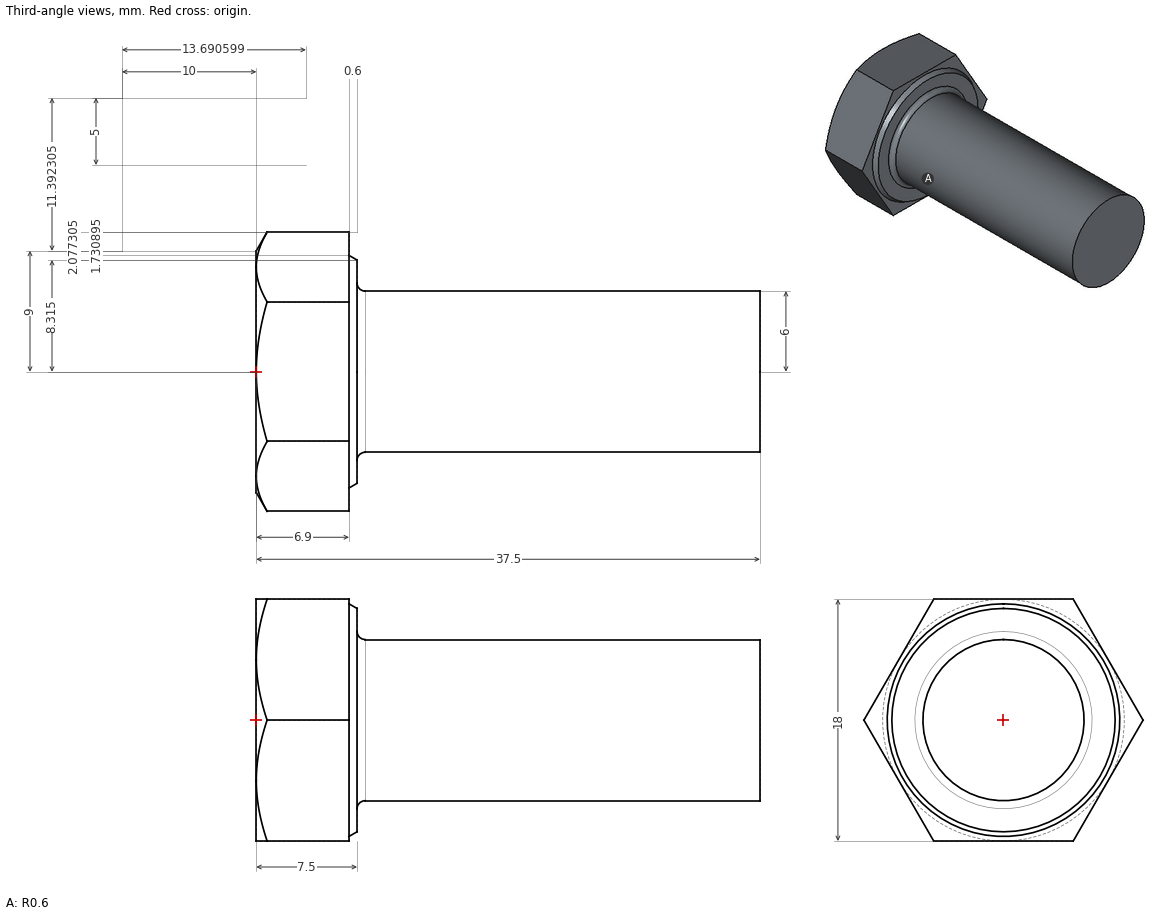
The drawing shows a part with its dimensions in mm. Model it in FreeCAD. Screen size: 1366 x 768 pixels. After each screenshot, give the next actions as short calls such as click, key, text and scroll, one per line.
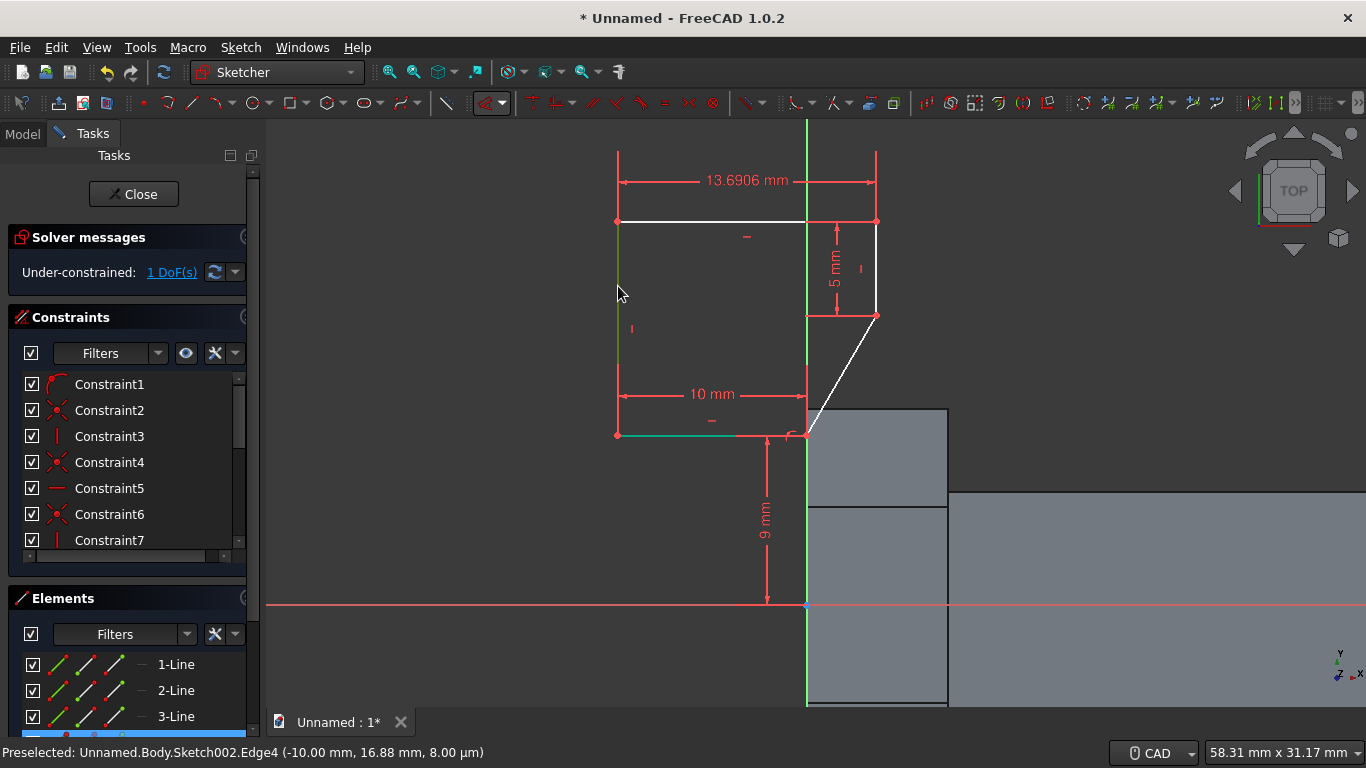
click(504, 104)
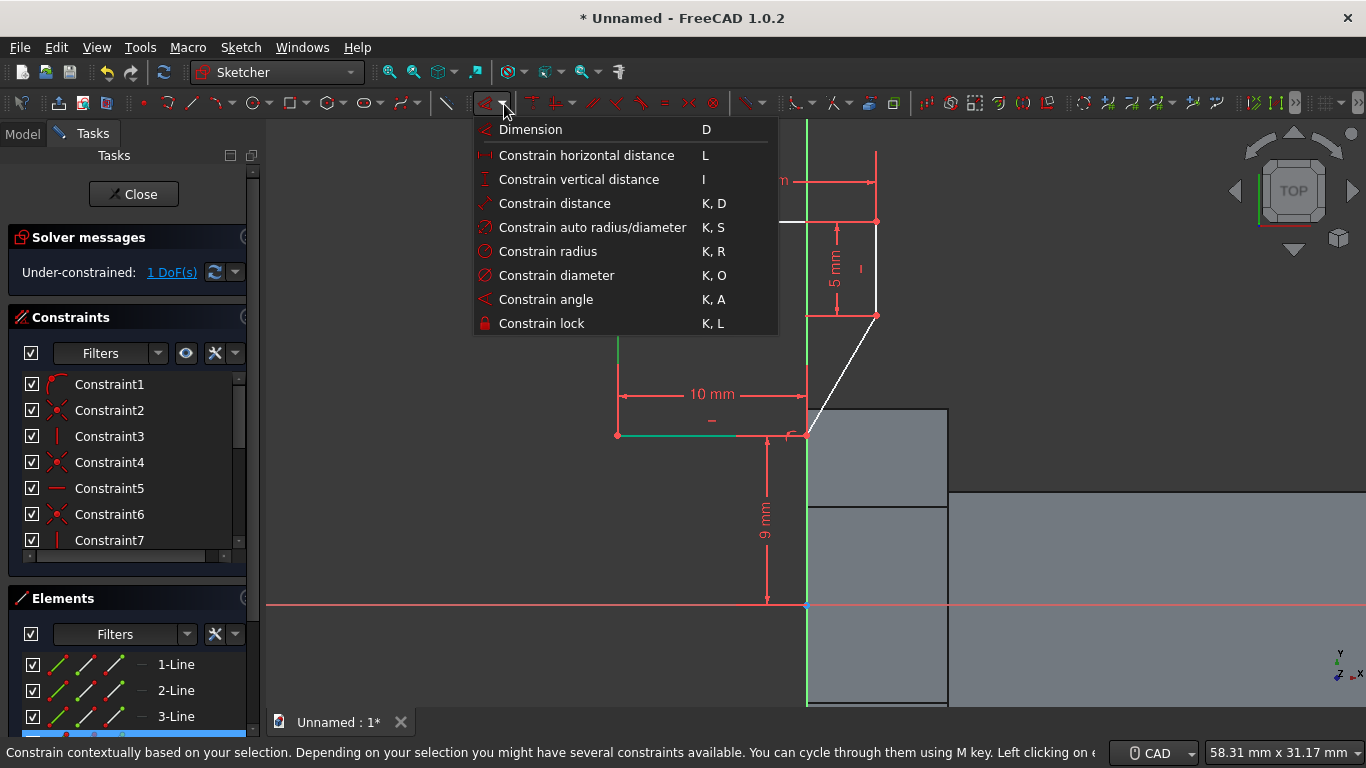
click(626, 179)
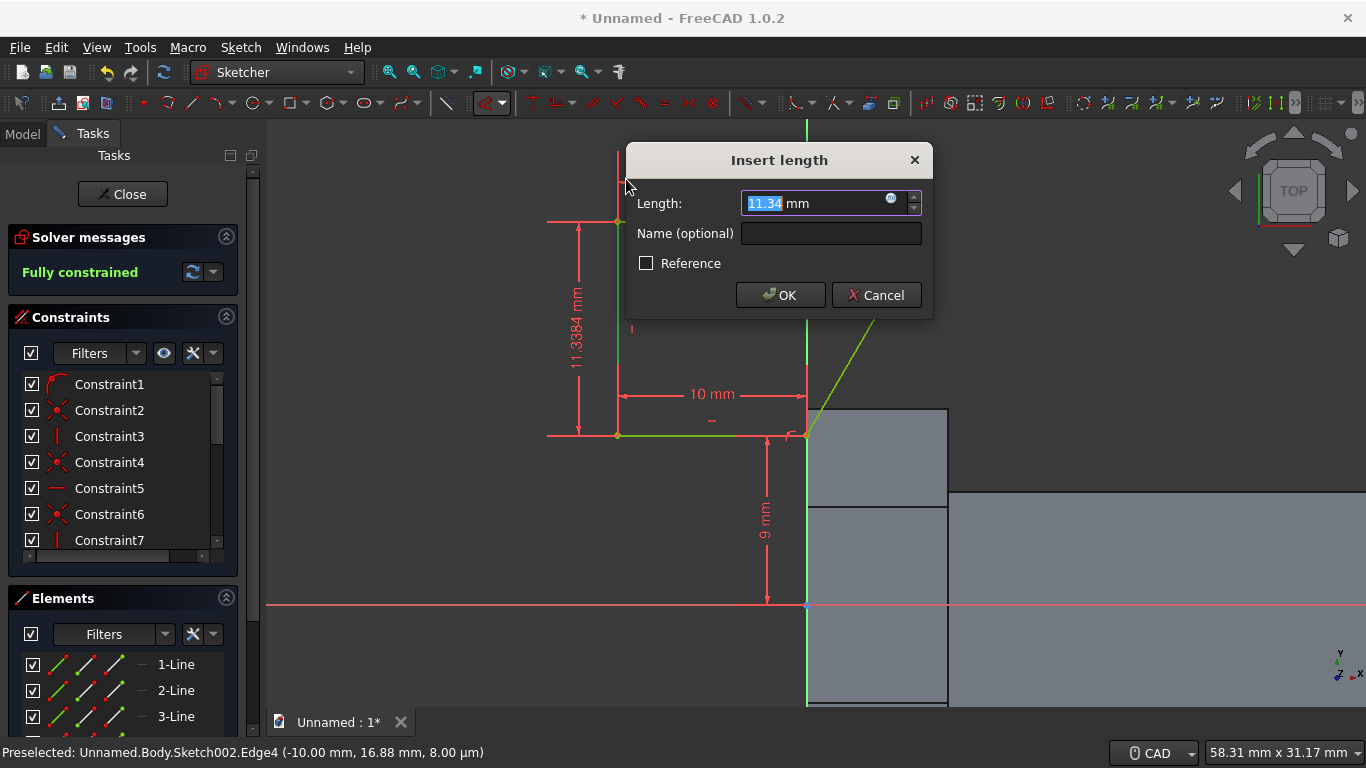
text(11.392305)
key(Return)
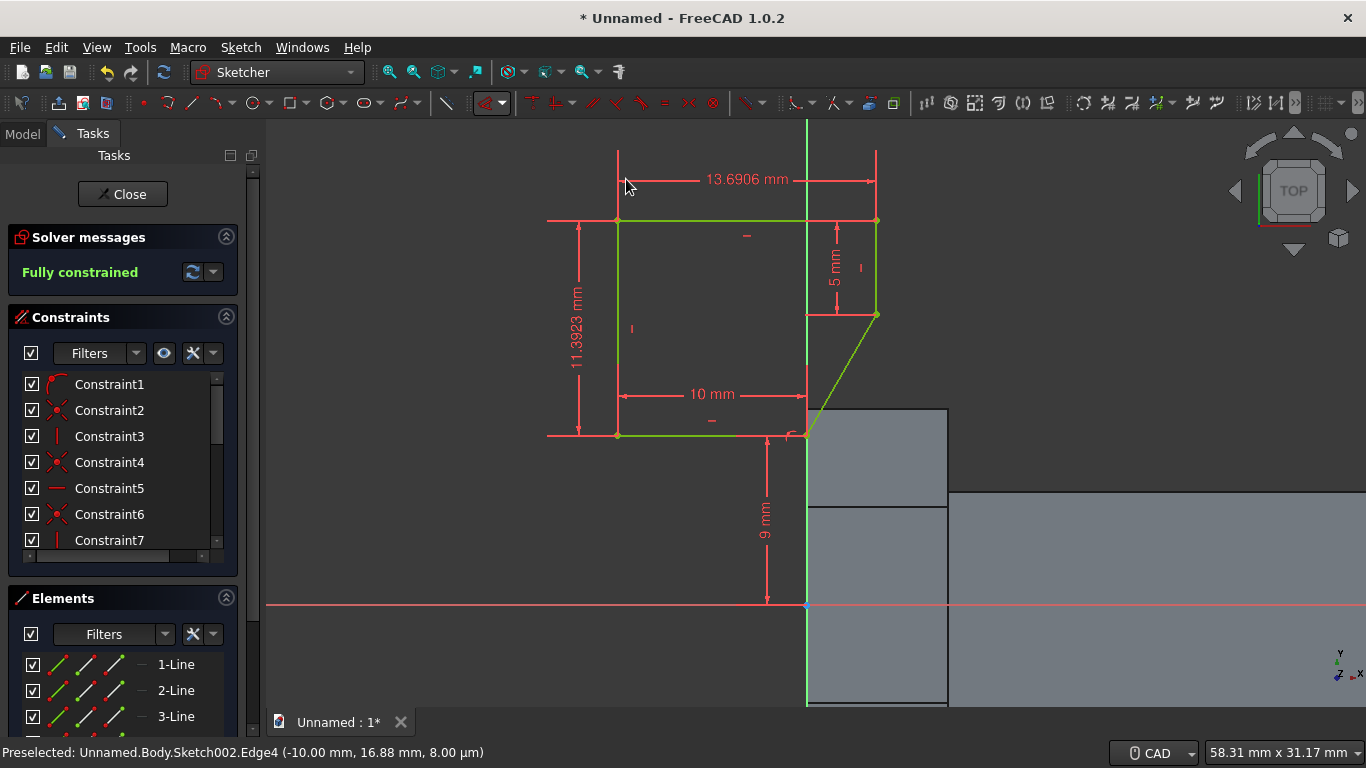
click(123, 194)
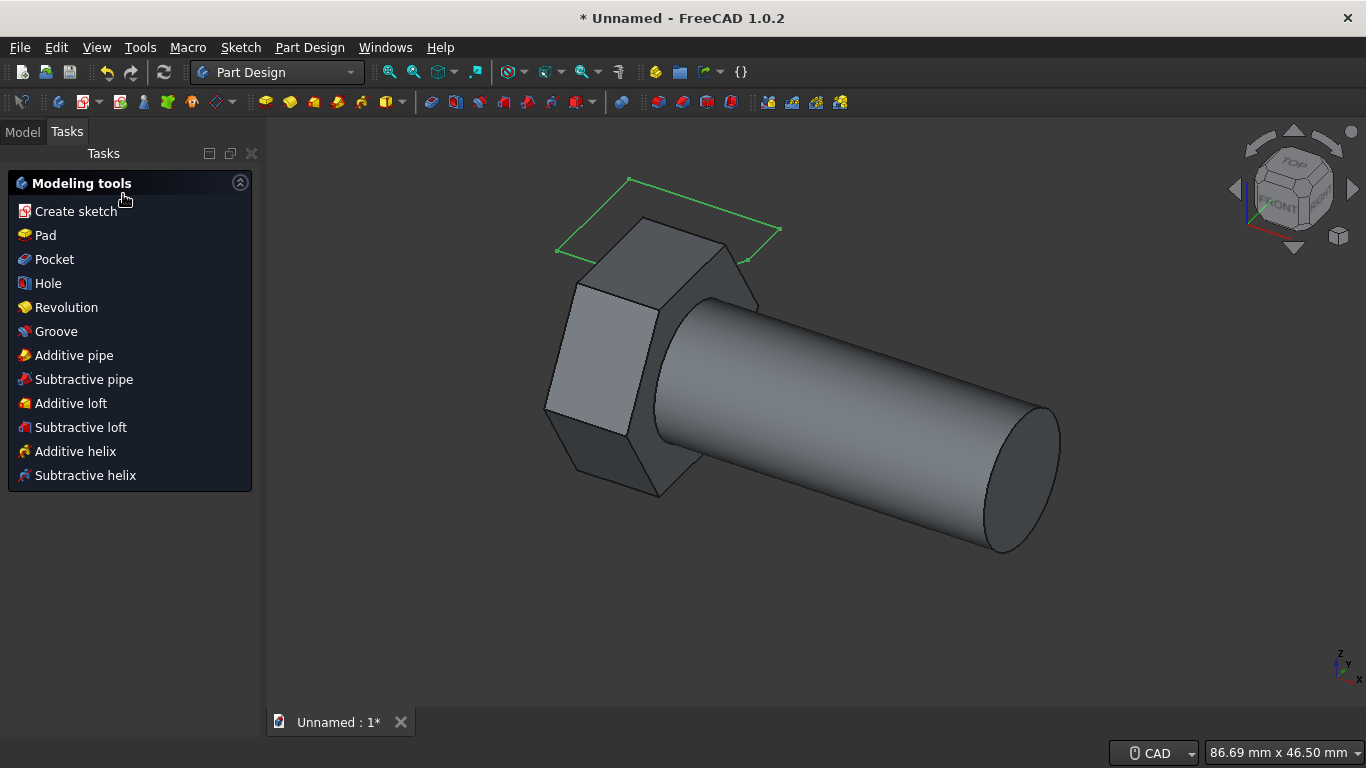
click(480, 102)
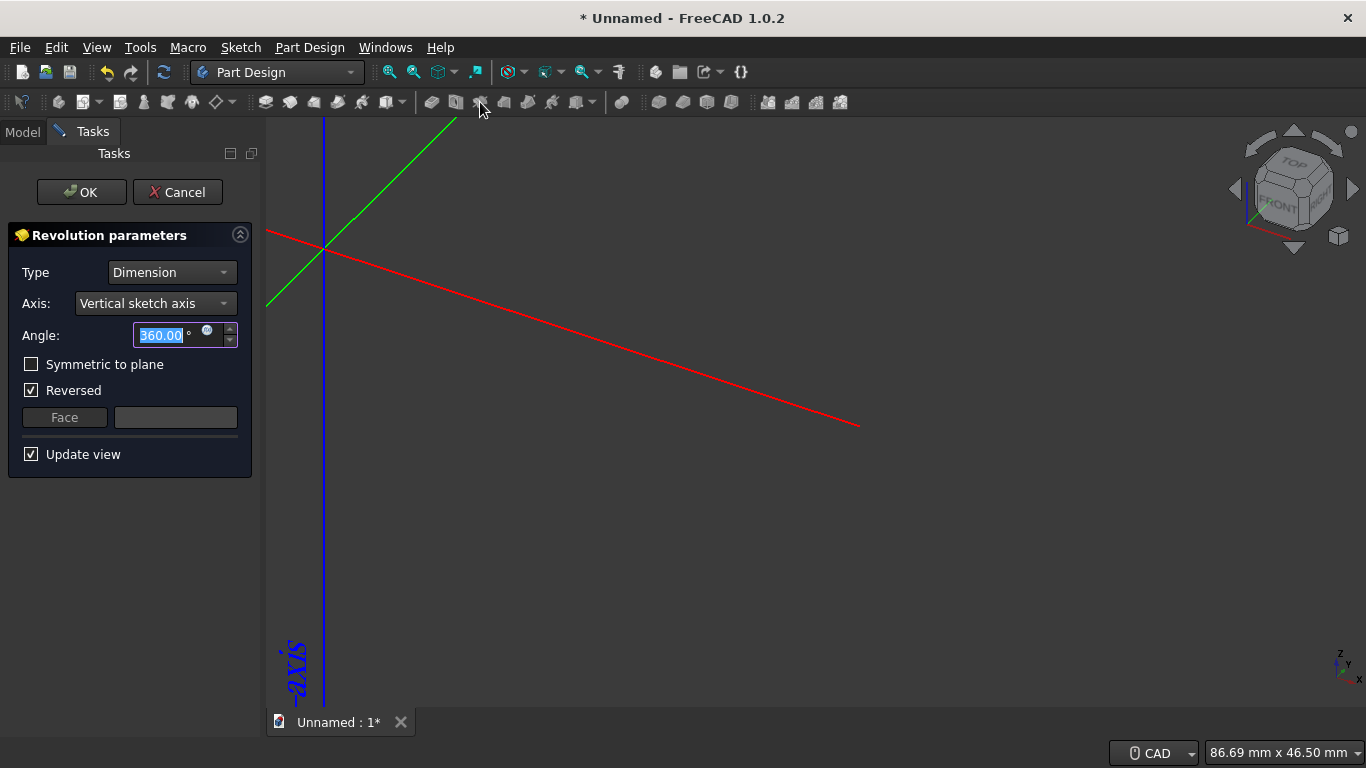
click(156, 304)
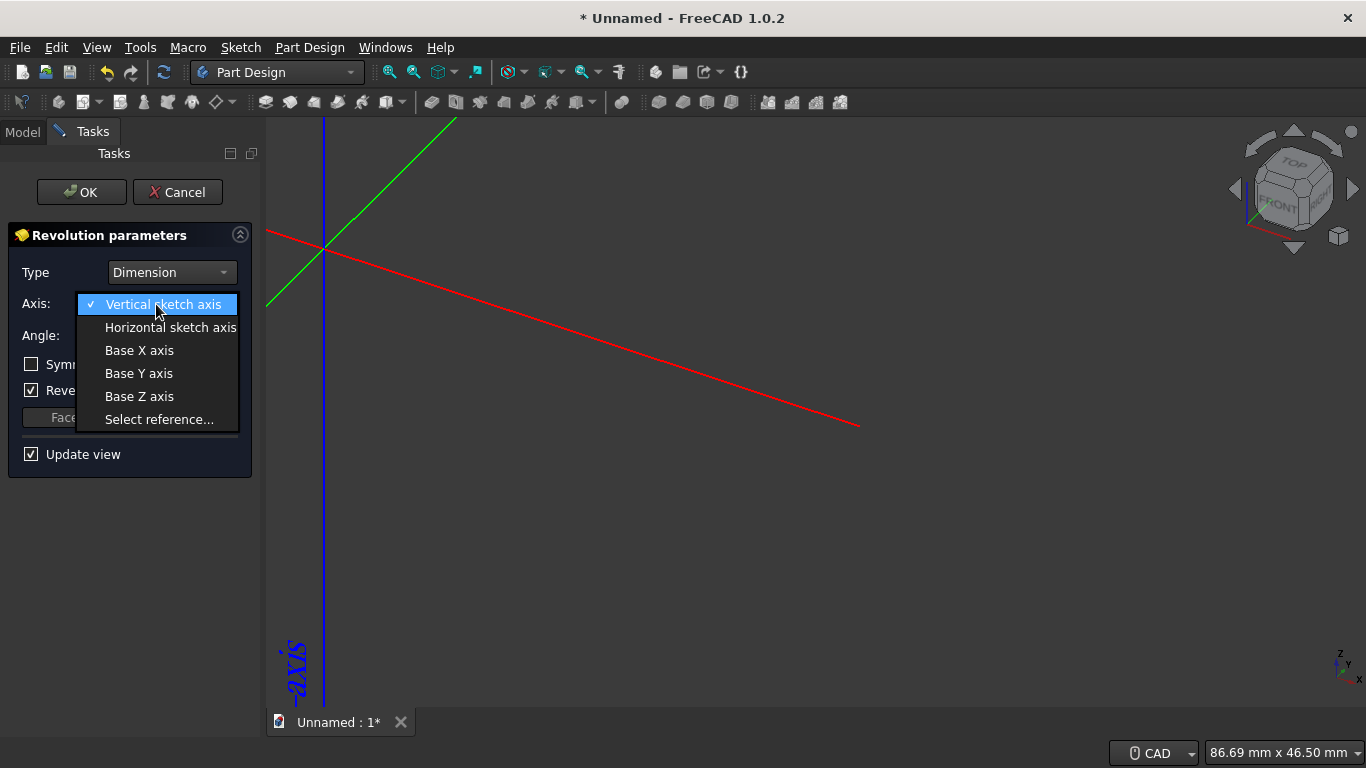
click(156, 328)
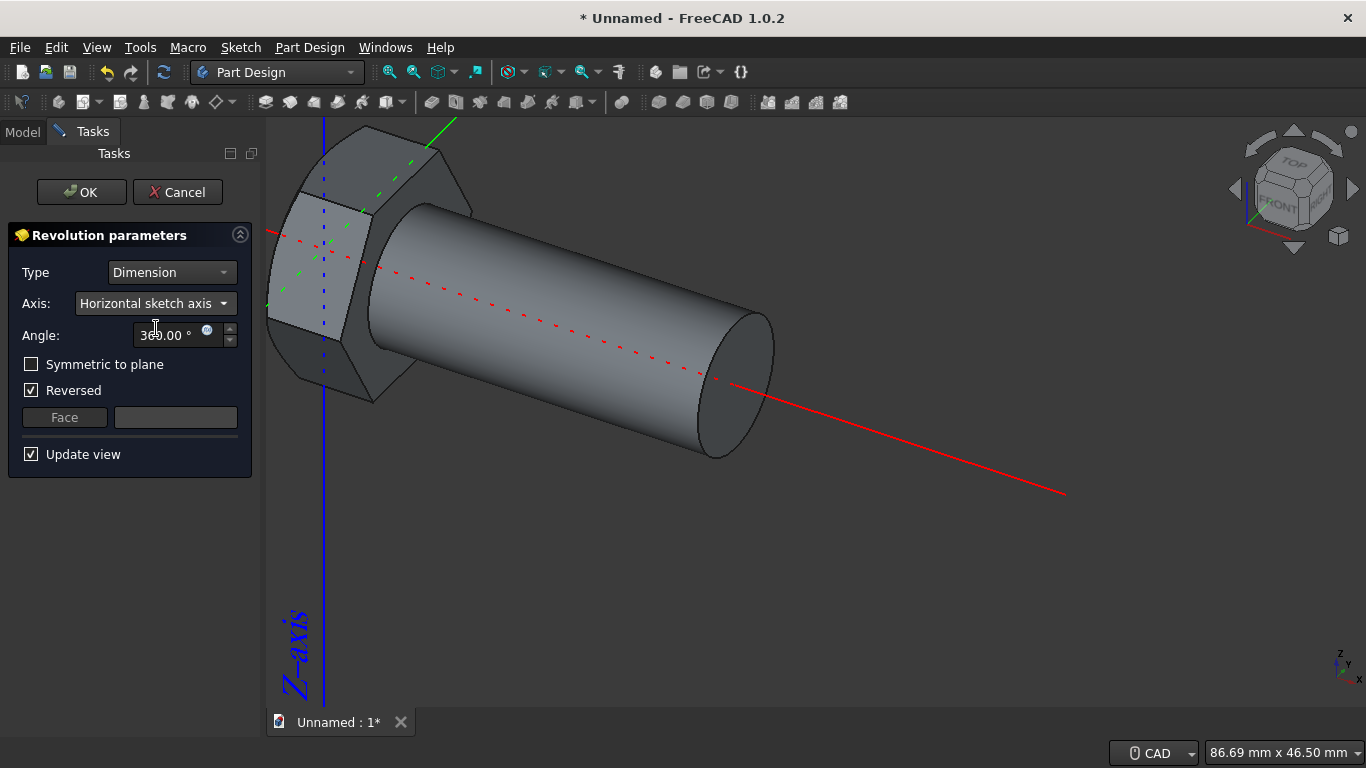
click(82, 192)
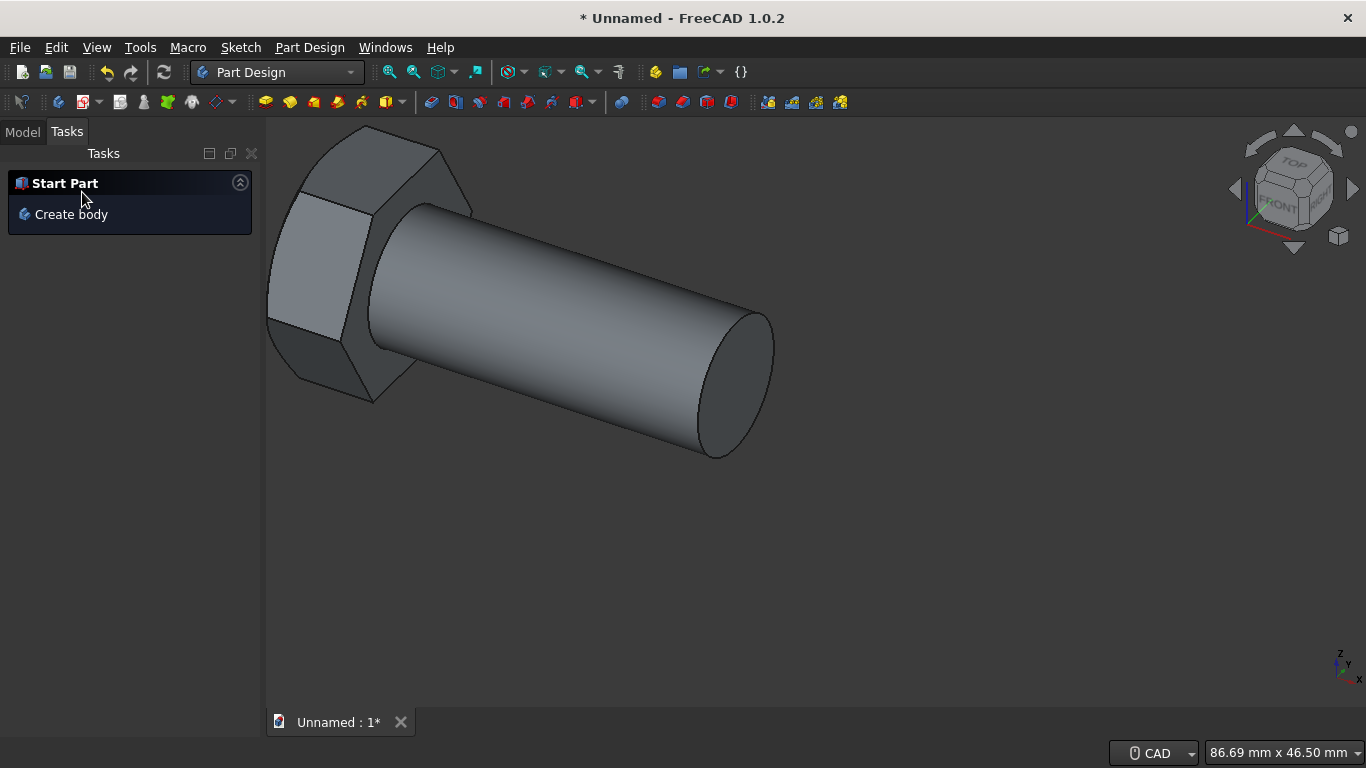
click(390, 72)